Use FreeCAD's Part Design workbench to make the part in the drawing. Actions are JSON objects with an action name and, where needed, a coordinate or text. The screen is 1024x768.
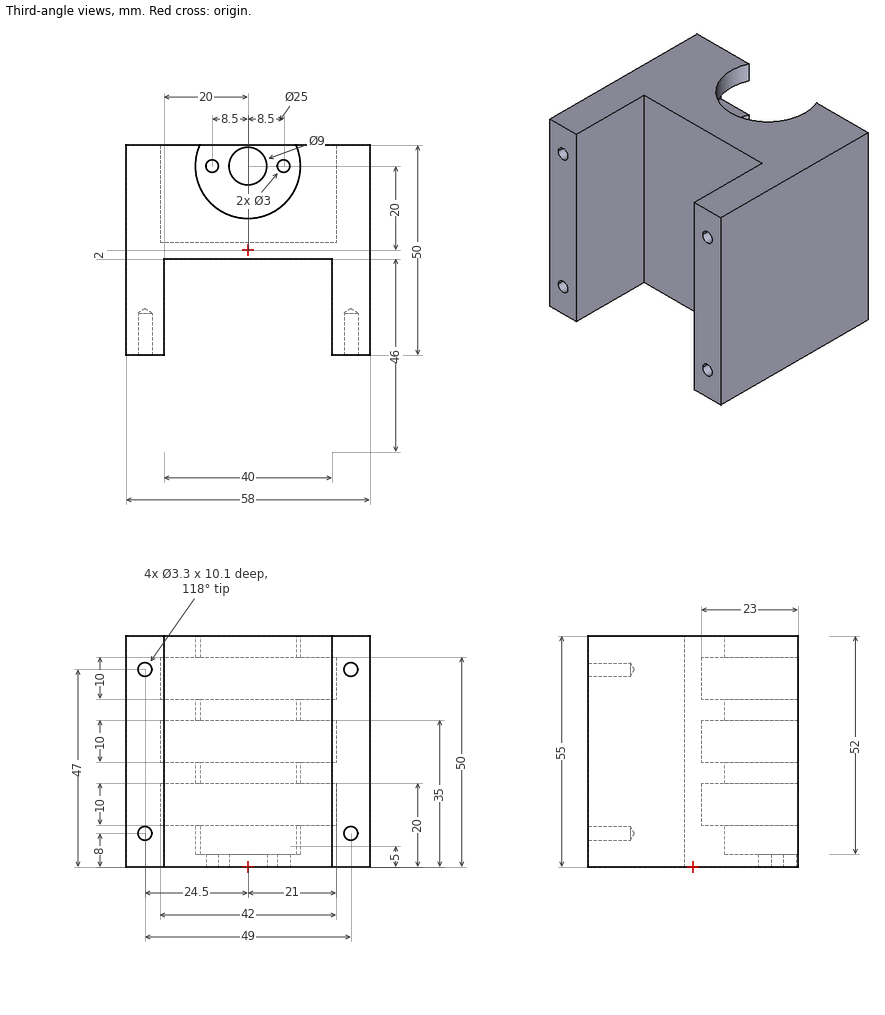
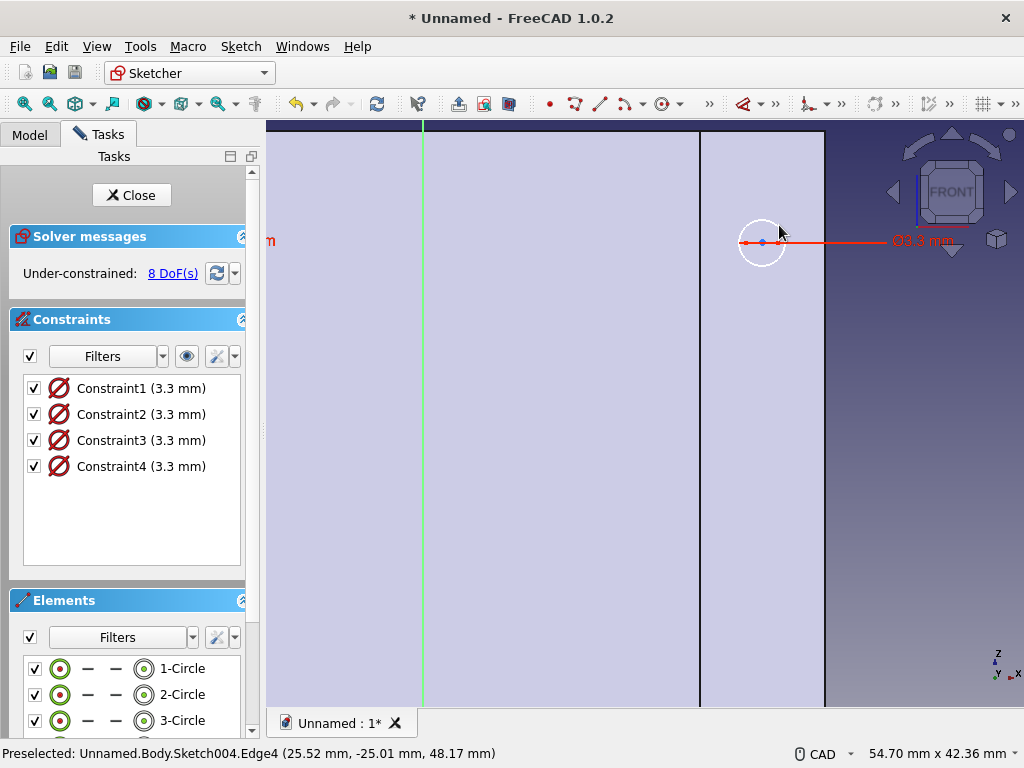
{"action": "left_click", "coordinate": [742, 104]}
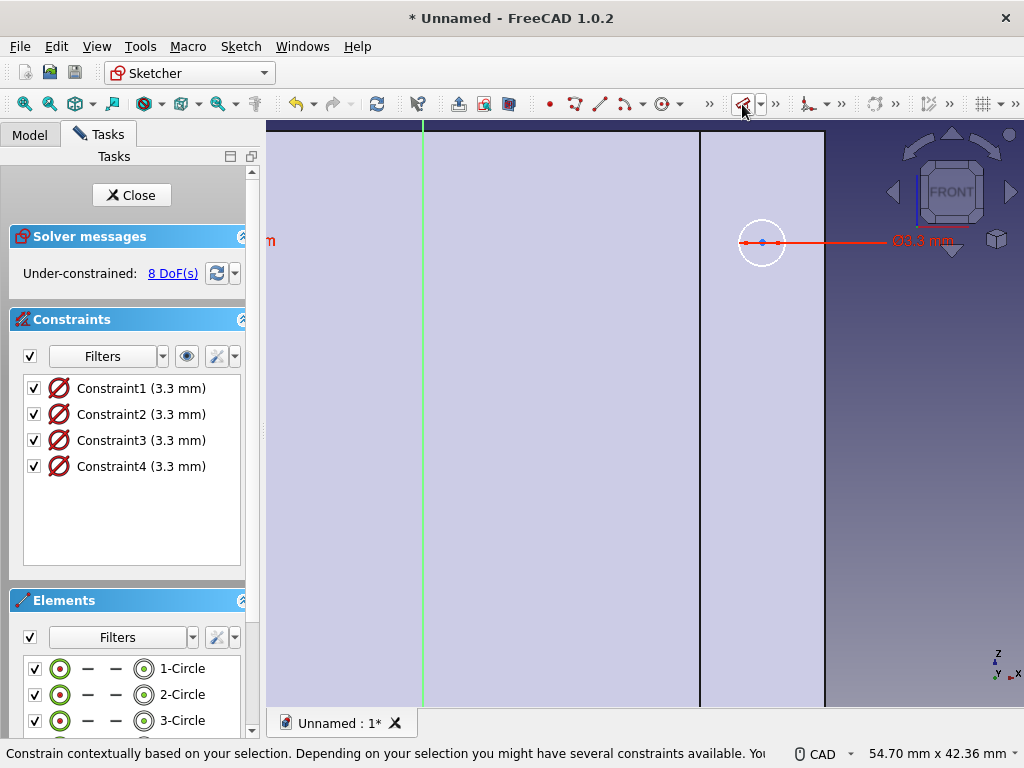
{"action": "scroll", "coordinate": [763, 240], "scroll_direction": "down", "scroll_amount": 3}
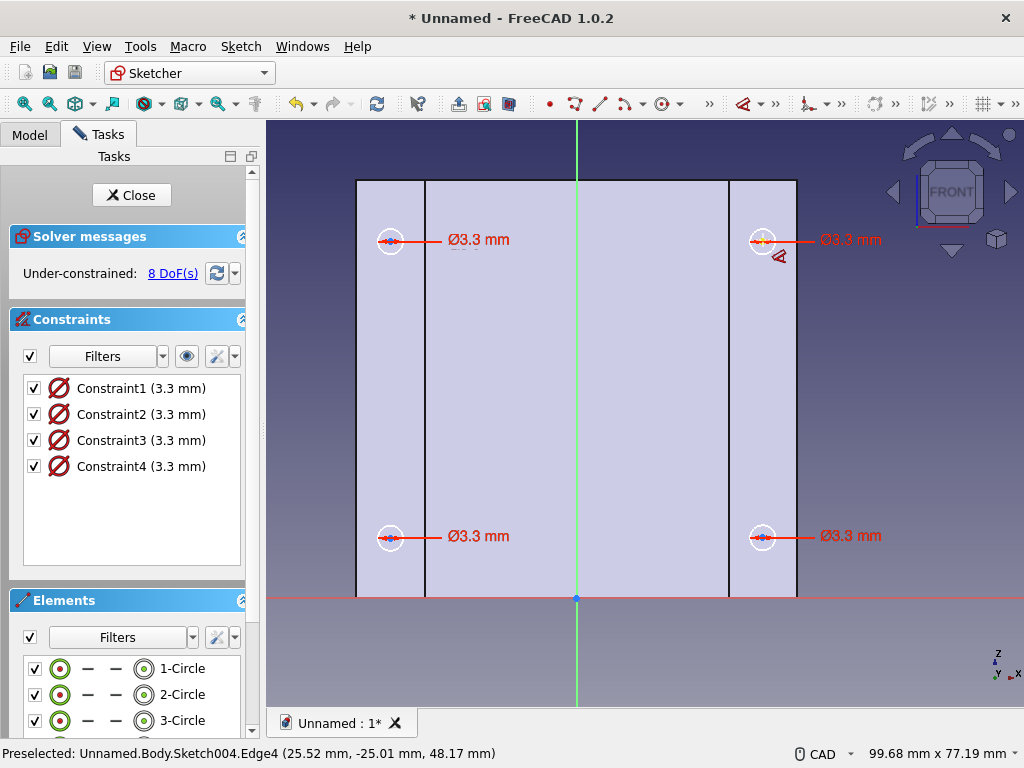
{"action": "left_click", "coordinate": [390, 538]}
{"action": "left_click", "coordinate": [356, 568]}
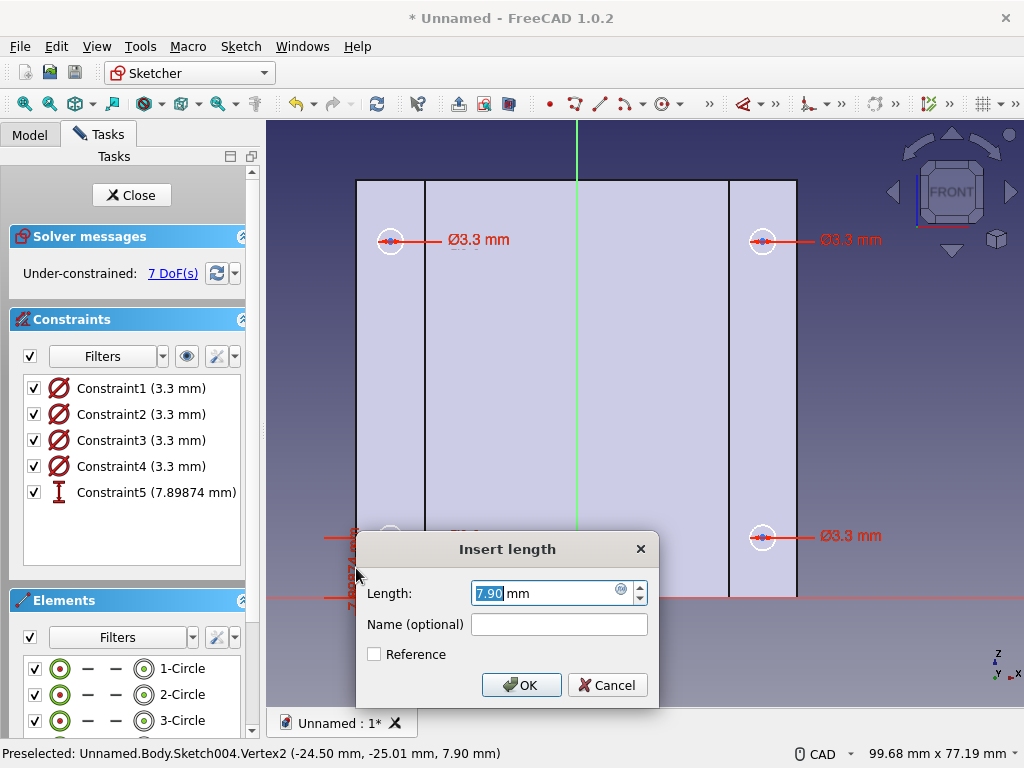
{"action": "type", "text": "8"}
{"action": "key", "text": "Return"}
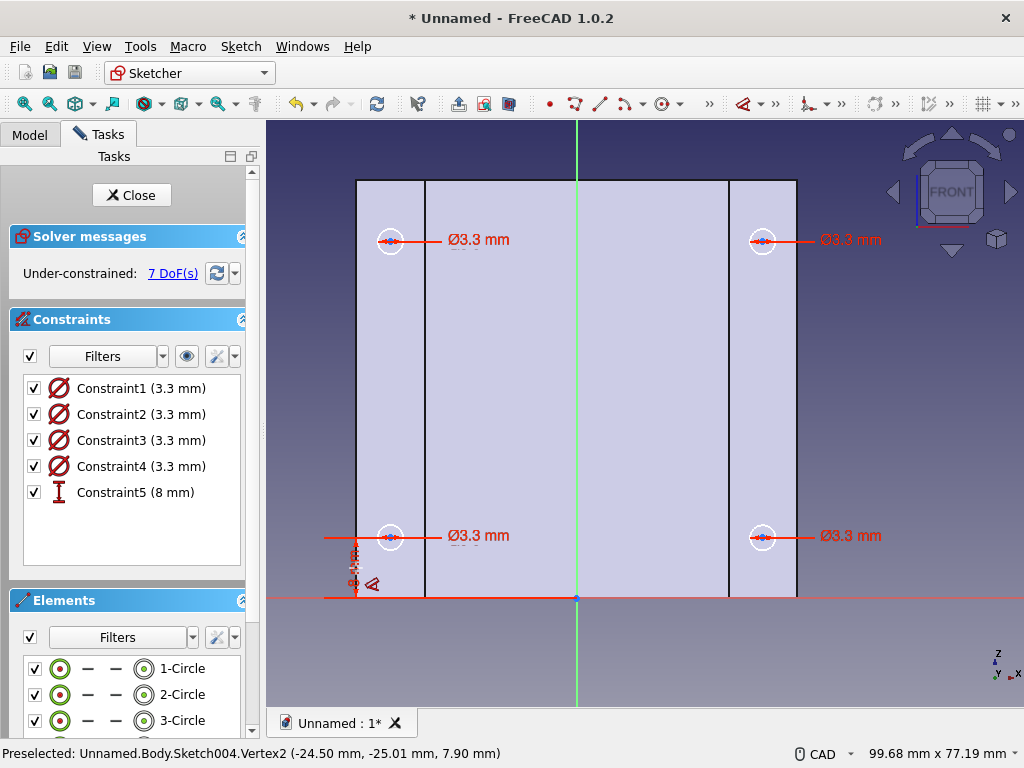
{"action": "left_click", "coordinate": [763, 538]}
{"action": "left_click", "coordinate": [797, 568]}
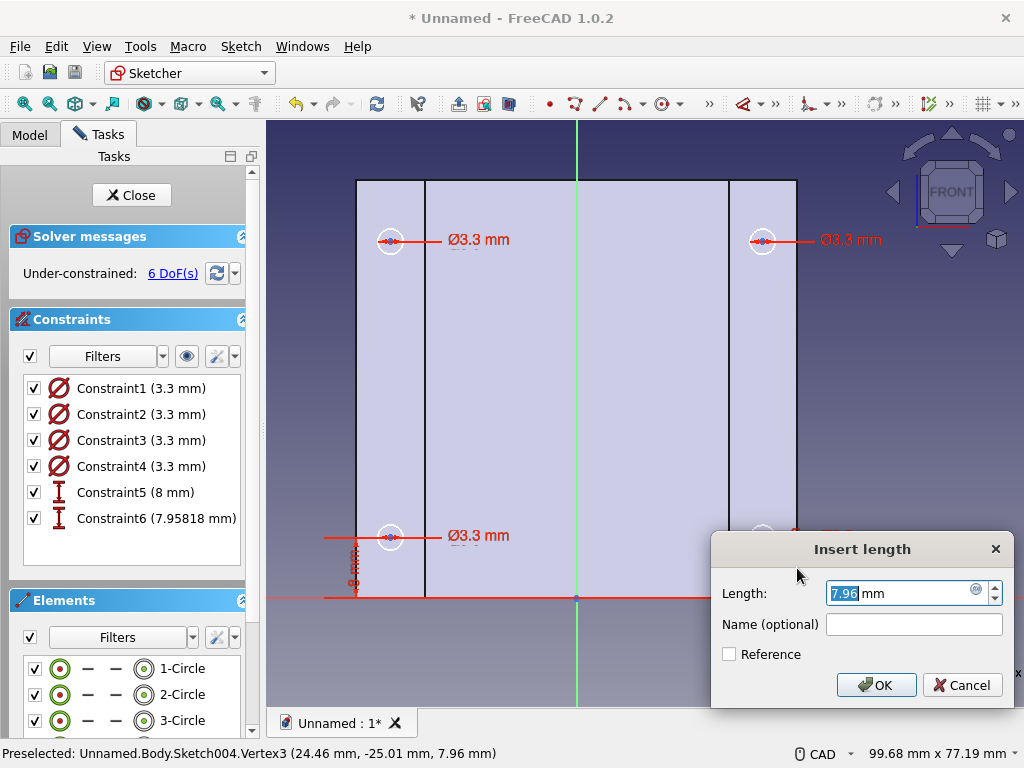
{"action": "type", "text": "8"}
{"action": "key", "text": "Return"}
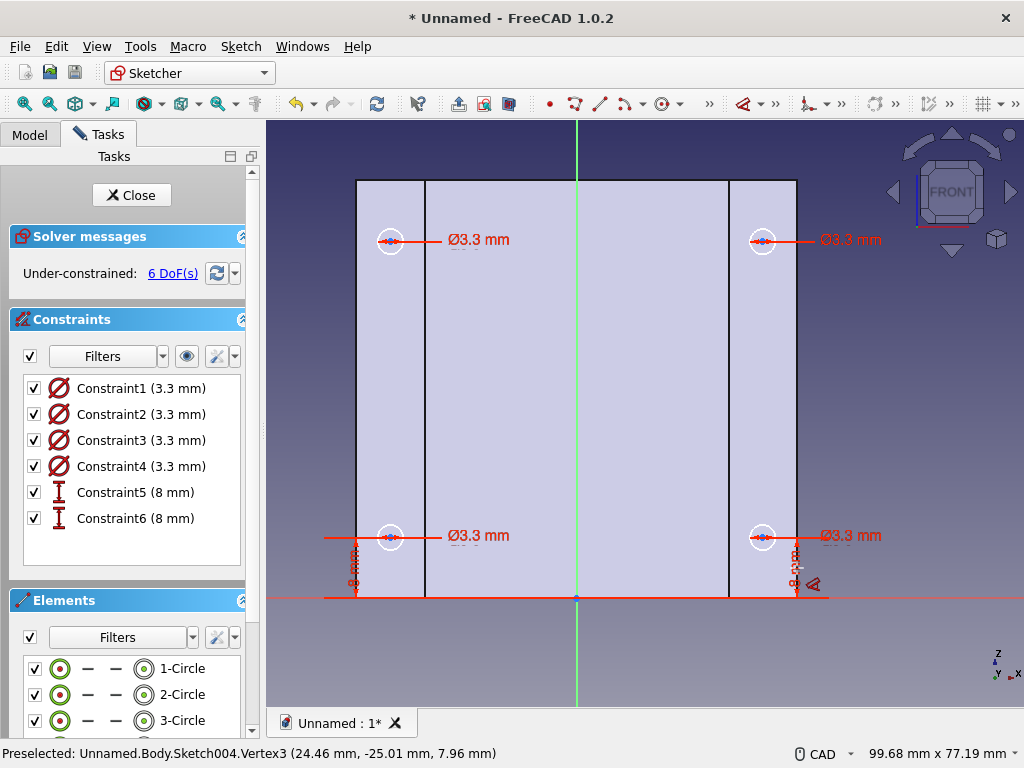
{"action": "left_click", "coordinate": [391, 242]}
{"action": "left_click", "coordinate": [357, 420]}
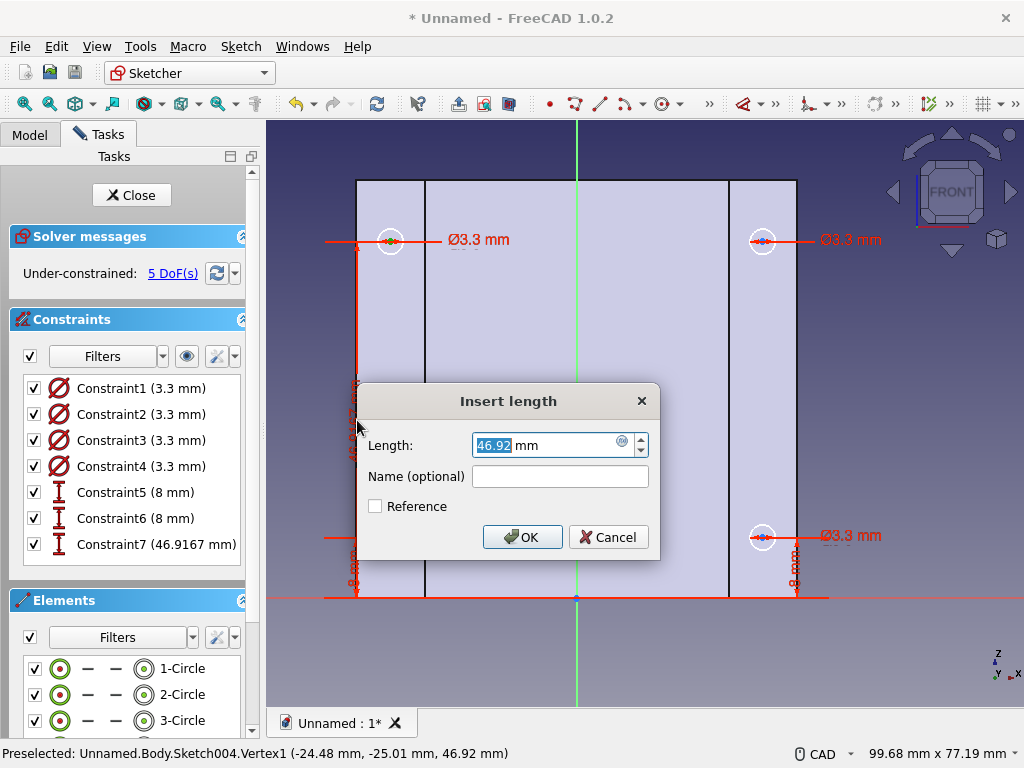
{"action": "type", "text": "47"}
{"action": "key", "text": "Return"}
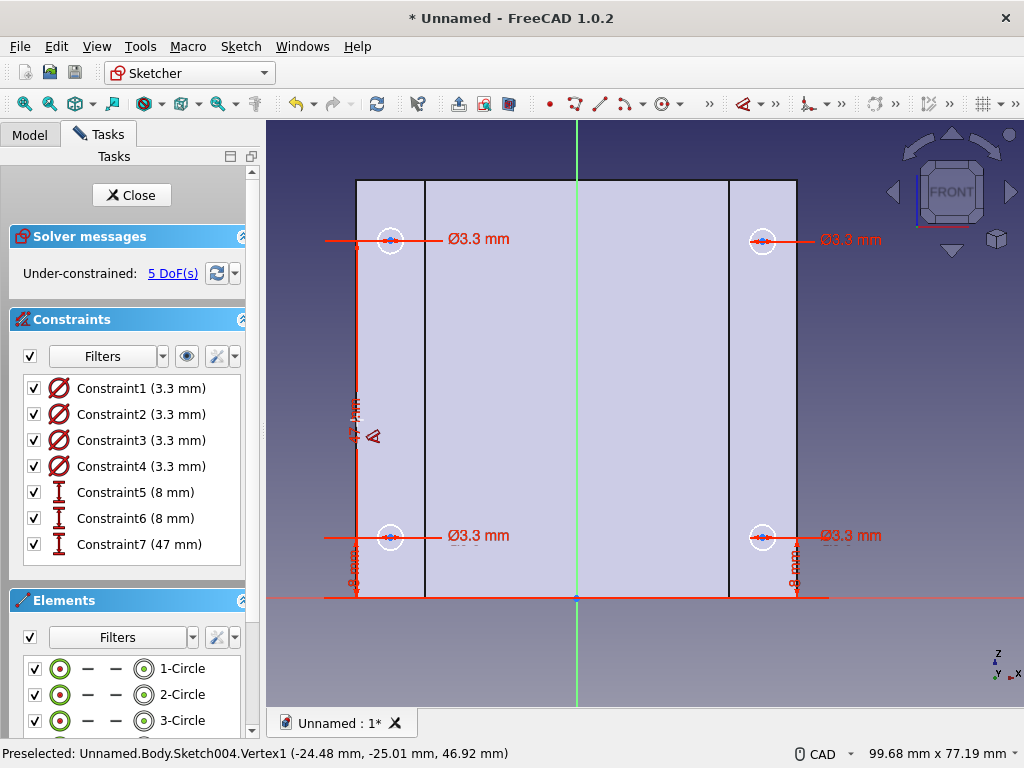
{"action": "left_click", "coordinate": [763, 242]}
{"action": "left_click", "coordinate": [797, 420]}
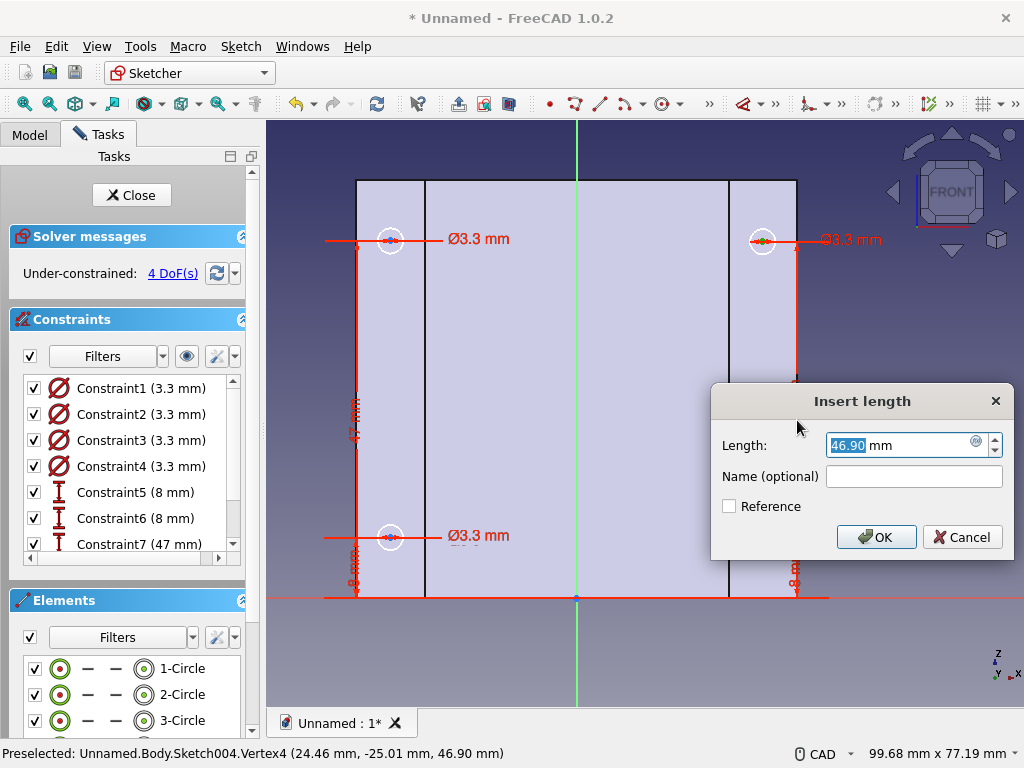
{"action": "type", "text": "47"}
{"action": "key", "text": "Return"}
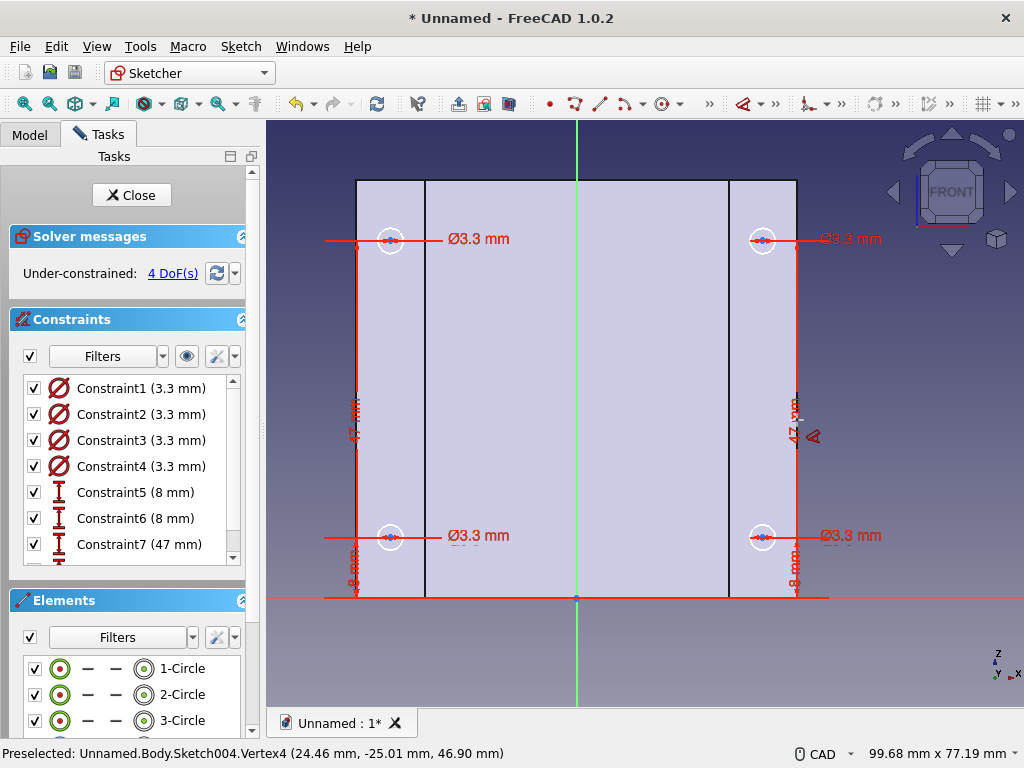
{"action": "left_click", "coordinate": [390, 538]}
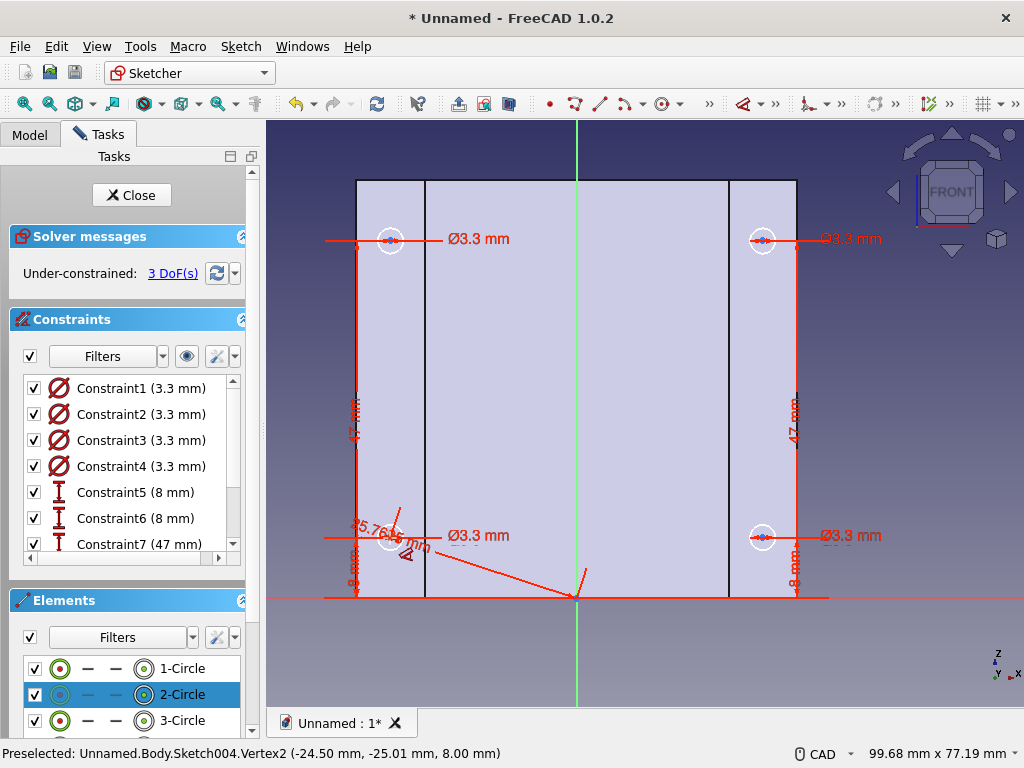
{"action": "left_click", "coordinate": [763, 538]}
{"action": "left_click", "coordinate": [491, 572]}